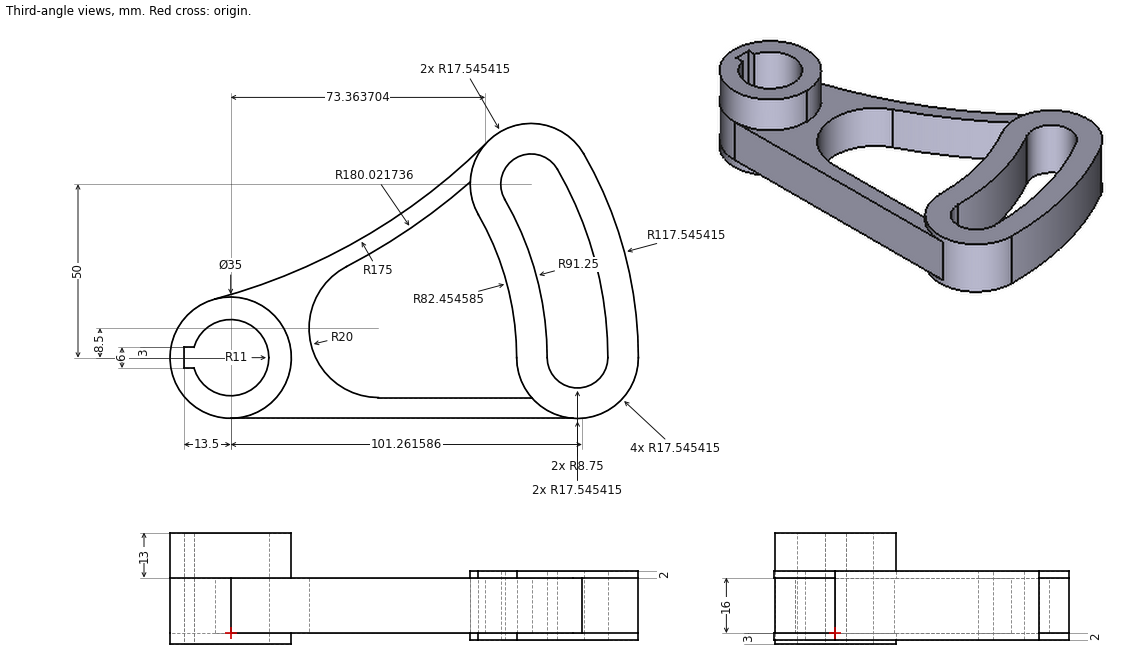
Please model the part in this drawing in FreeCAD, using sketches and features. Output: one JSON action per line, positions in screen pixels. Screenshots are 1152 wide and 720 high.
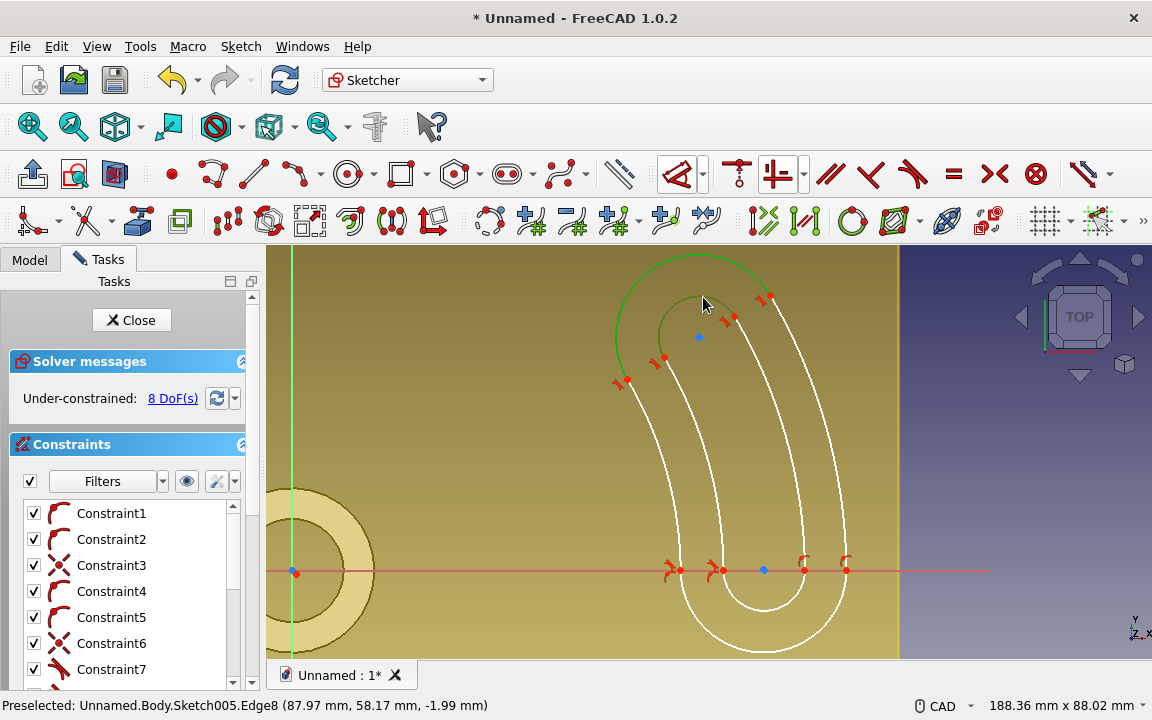
{"action": "left_click", "coordinate": [737, 174]}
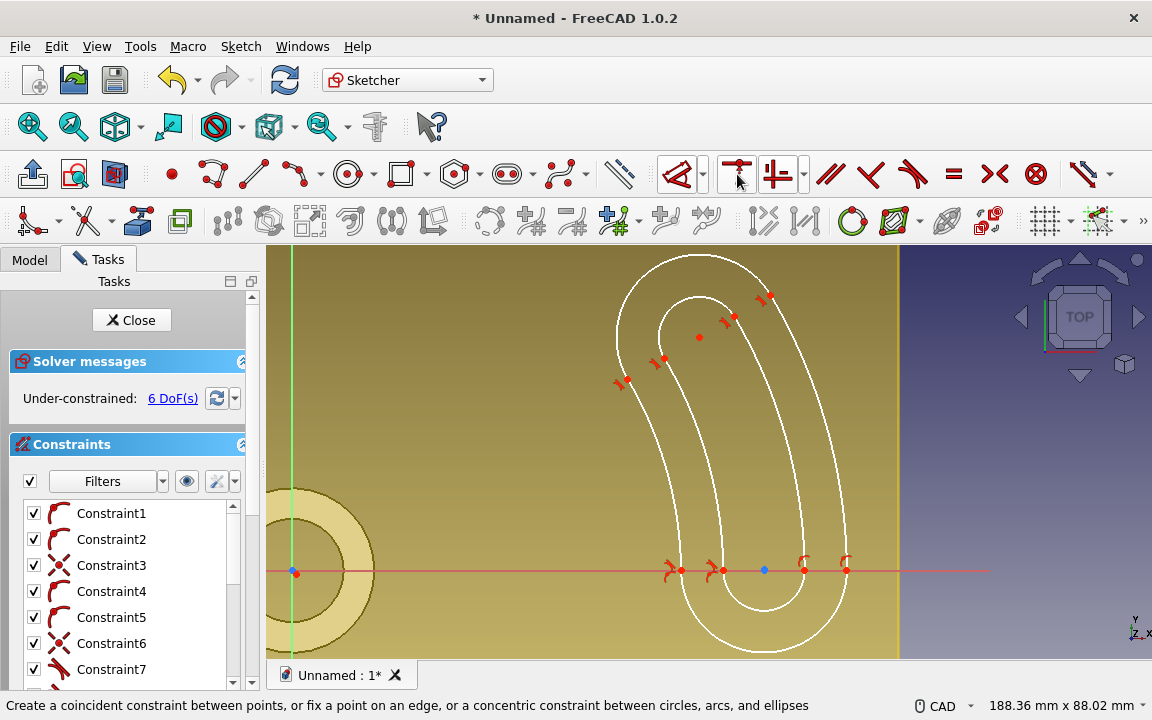
{"action": "left_click_drag", "start_coordinate": [282, 561], "coordinate": [306, 585]}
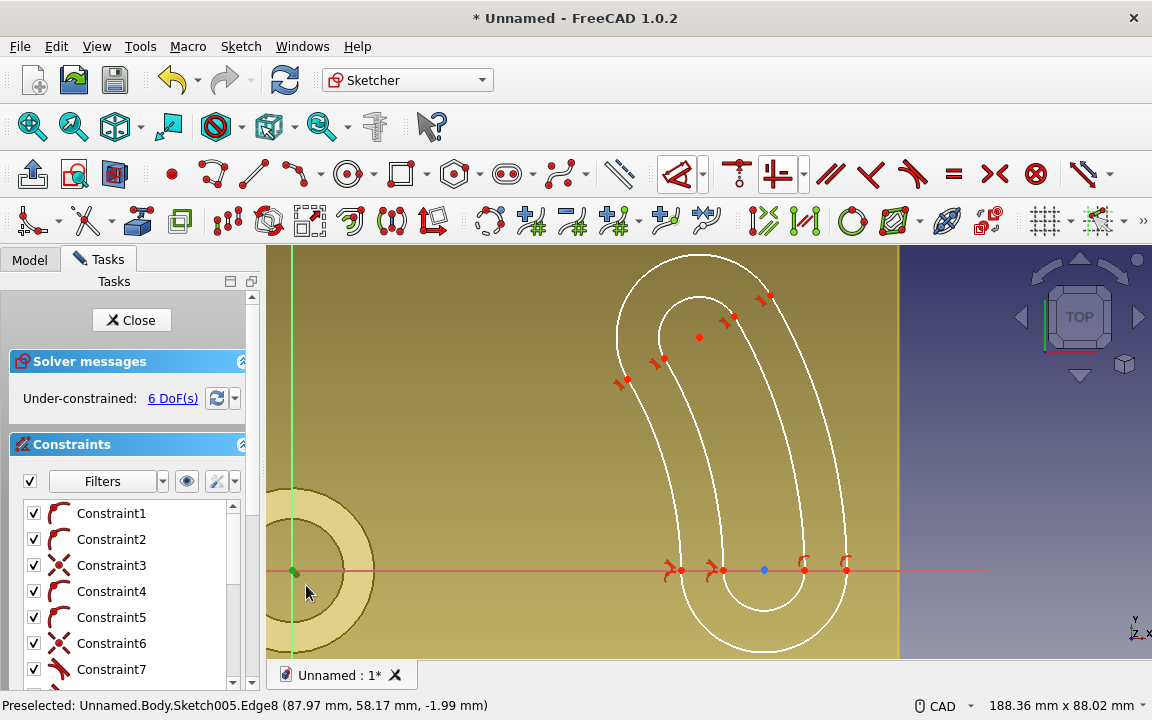
{"action": "left_click", "coordinate": [737, 174]}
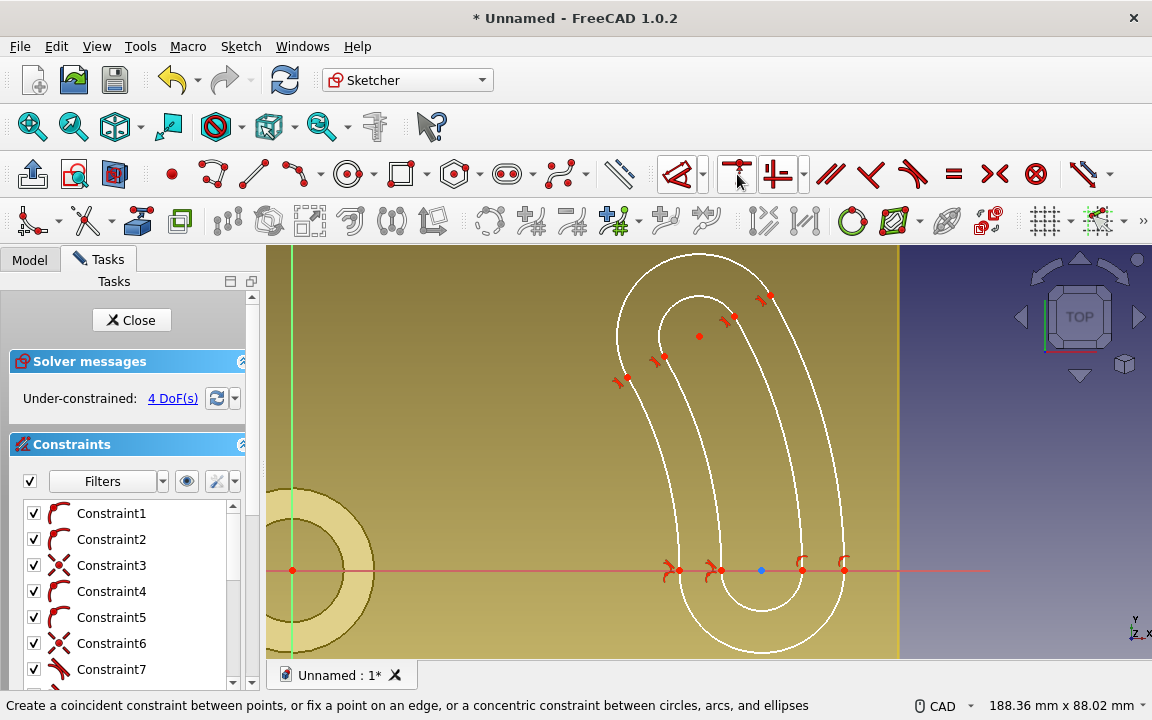
{"action": "left_click", "coordinate": [675, 510]}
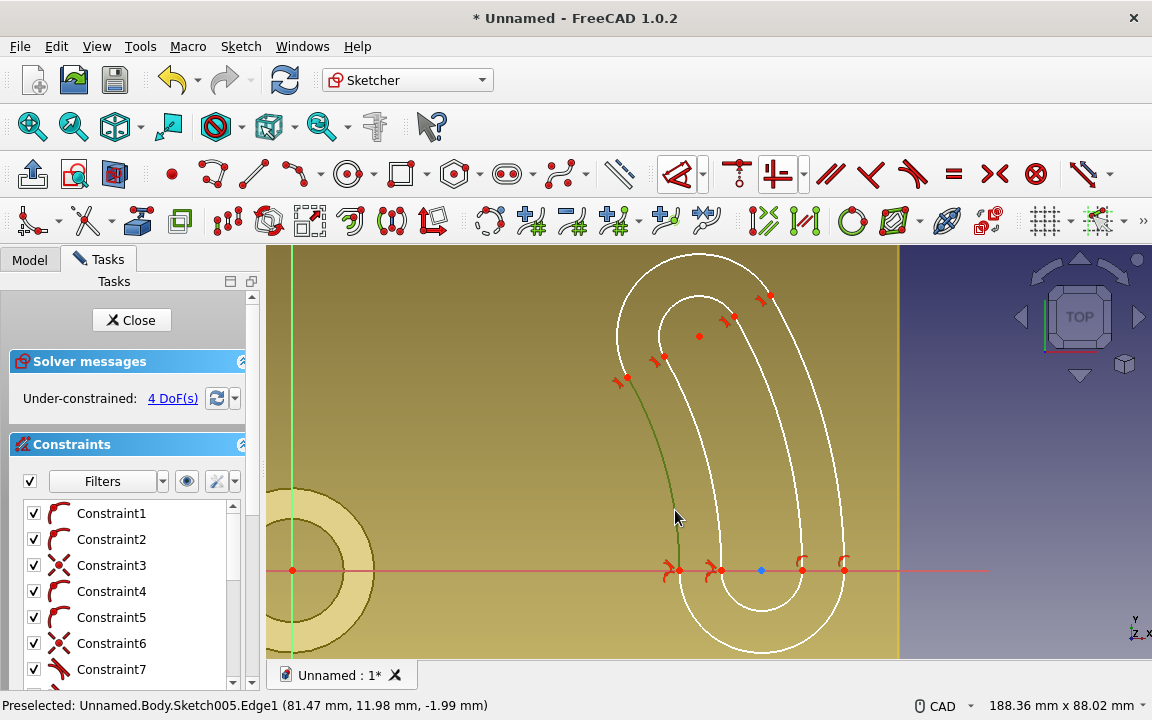
{"action": "key", "text": "k r"}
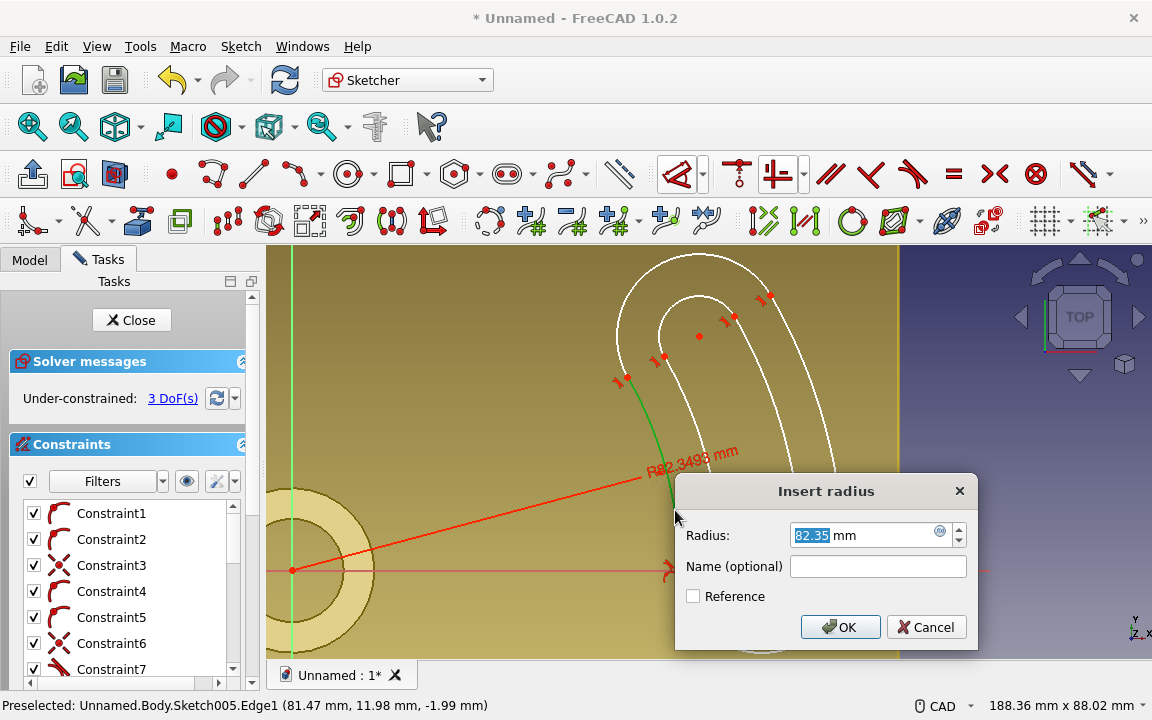
{"action": "type", "text": "82.454585"}
{"action": "key", "text": "Return"}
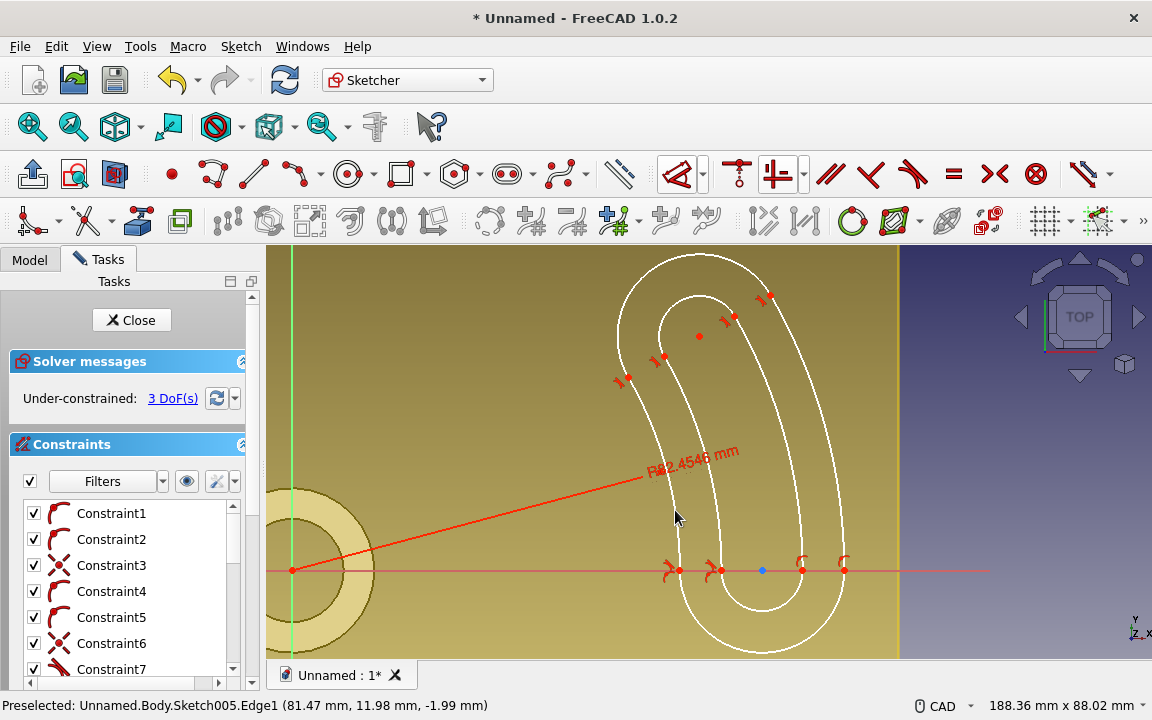
{"action": "left_click", "coordinate": [625, 303]}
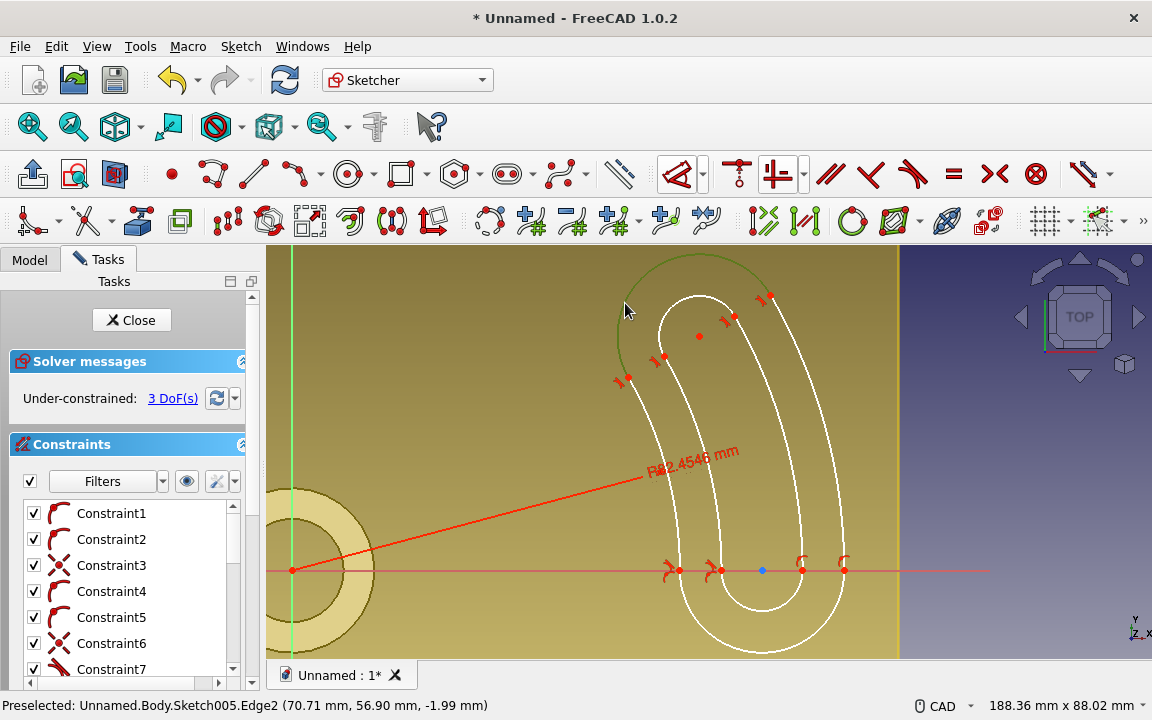
{"action": "key", "text": "k r"}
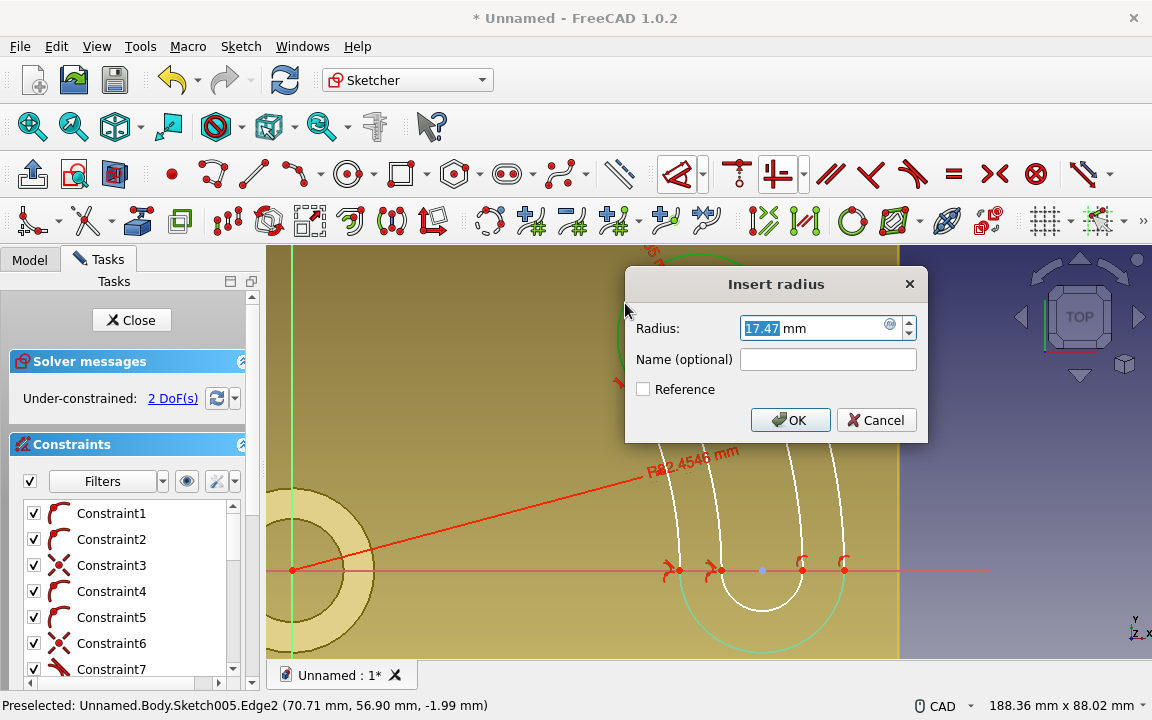
{"action": "type", "text": "17.545415"}
{"action": "key", "text": "Return"}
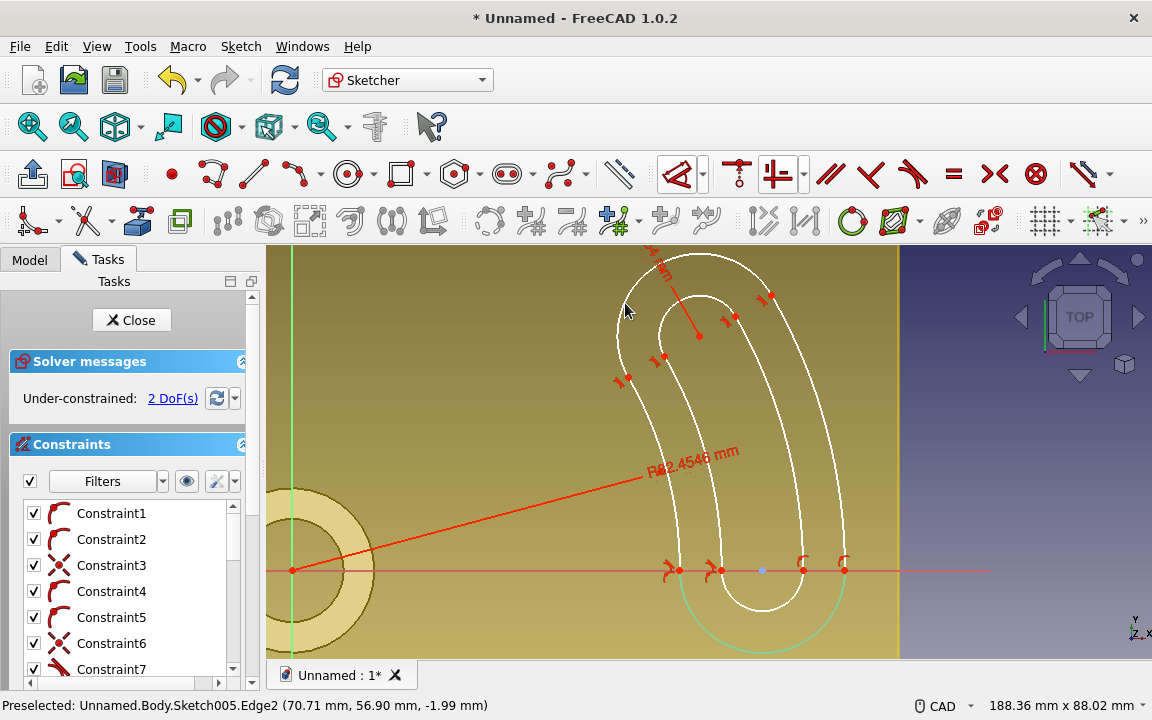
{"action": "left_click", "coordinate": [717, 504]}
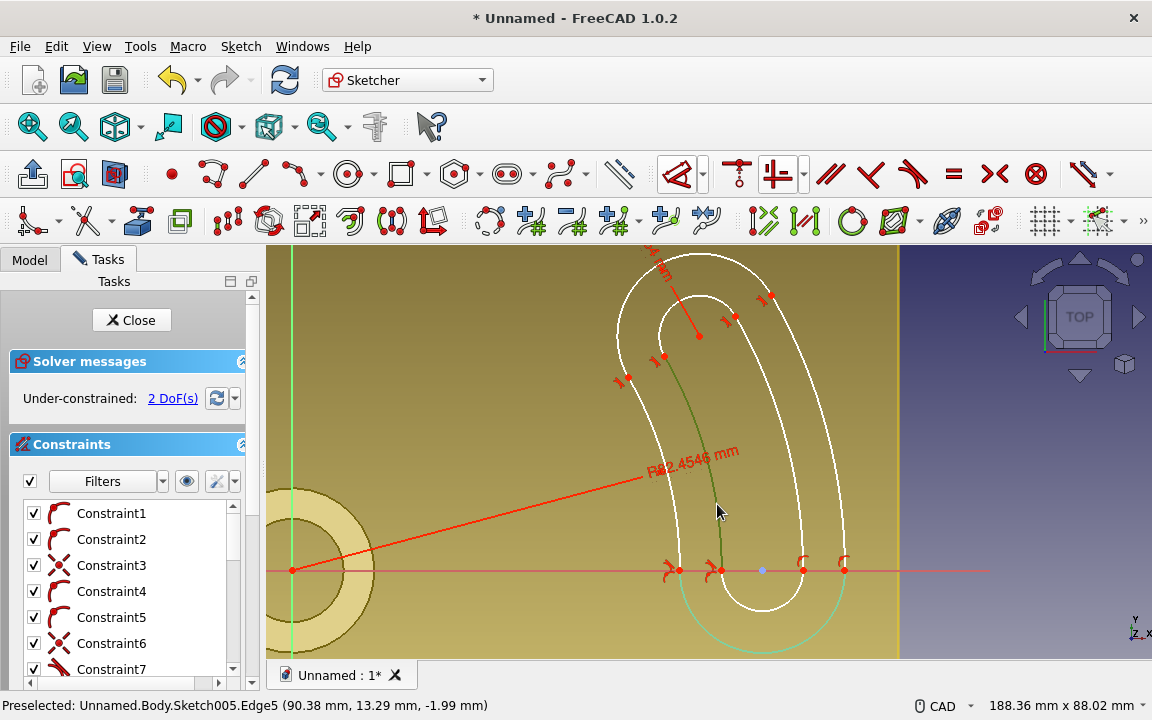
{"action": "left_click", "coordinate": [702, 174]}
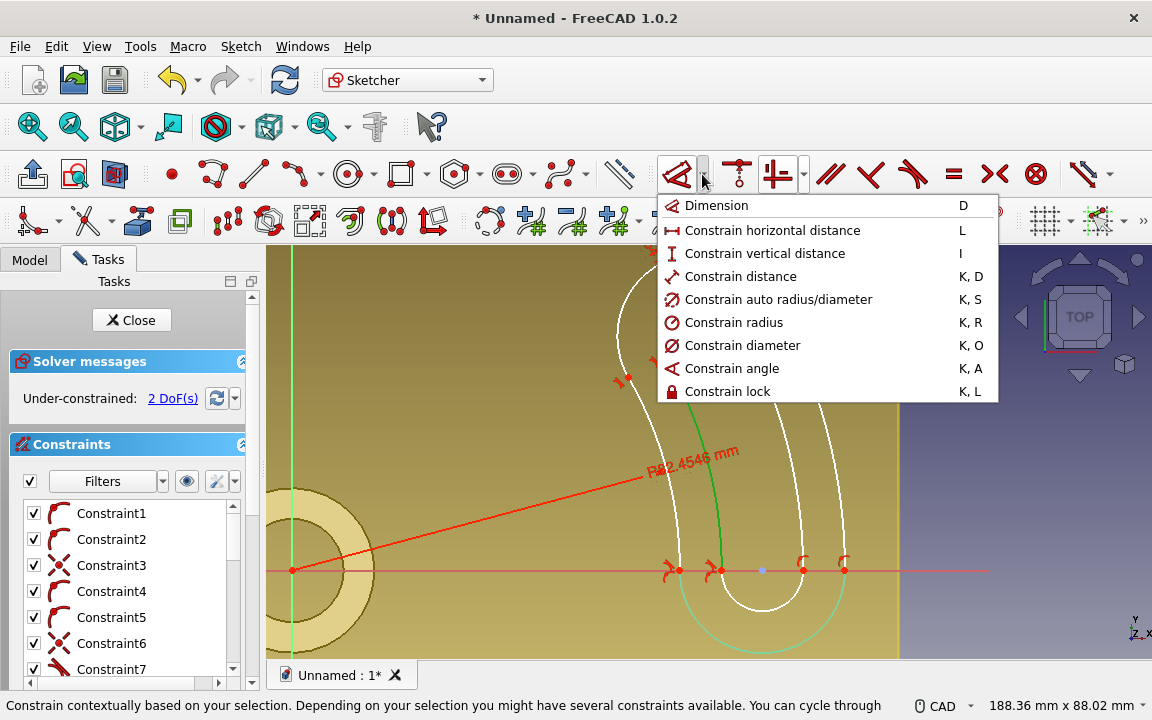
{"action": "left_click", "coordinate": [828, 322]}